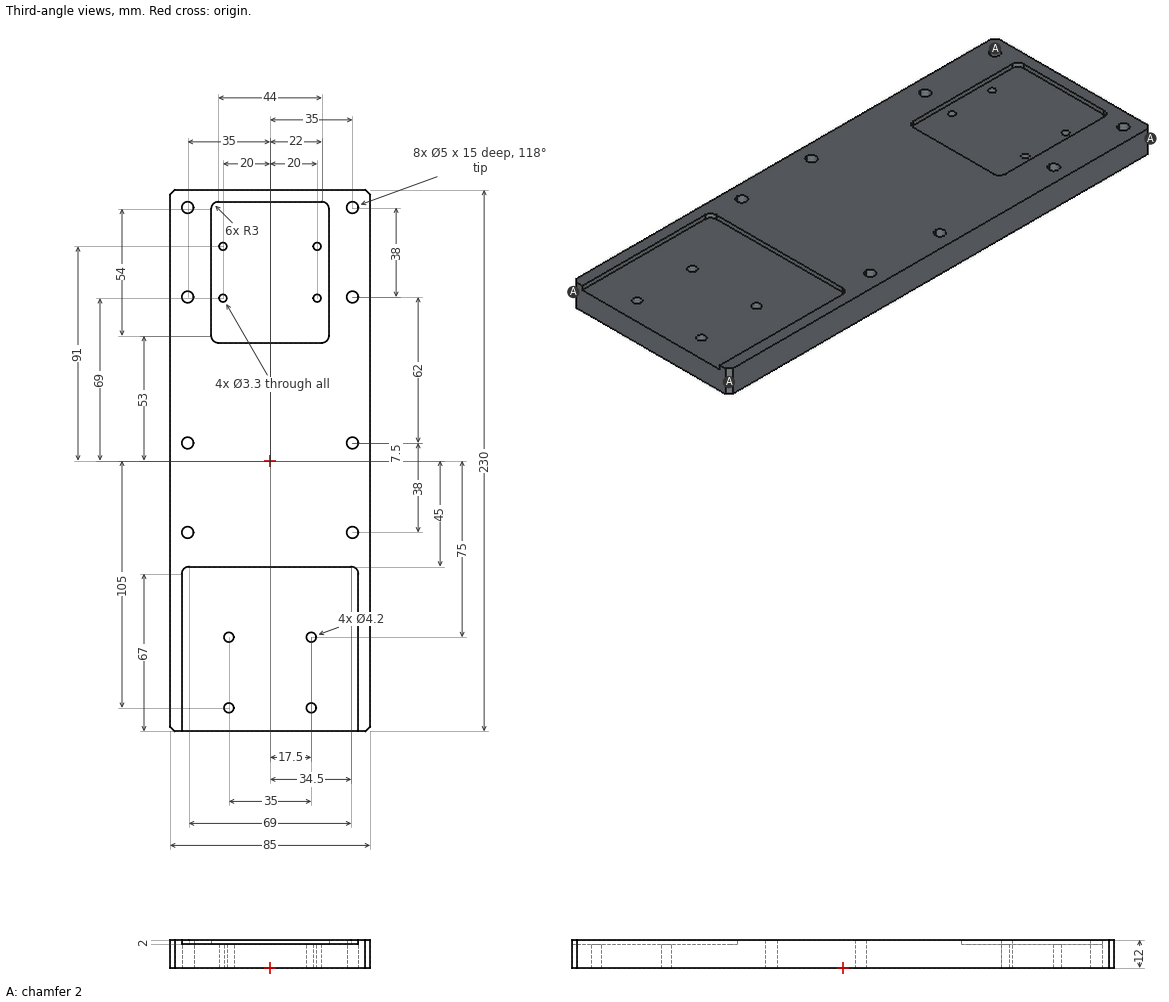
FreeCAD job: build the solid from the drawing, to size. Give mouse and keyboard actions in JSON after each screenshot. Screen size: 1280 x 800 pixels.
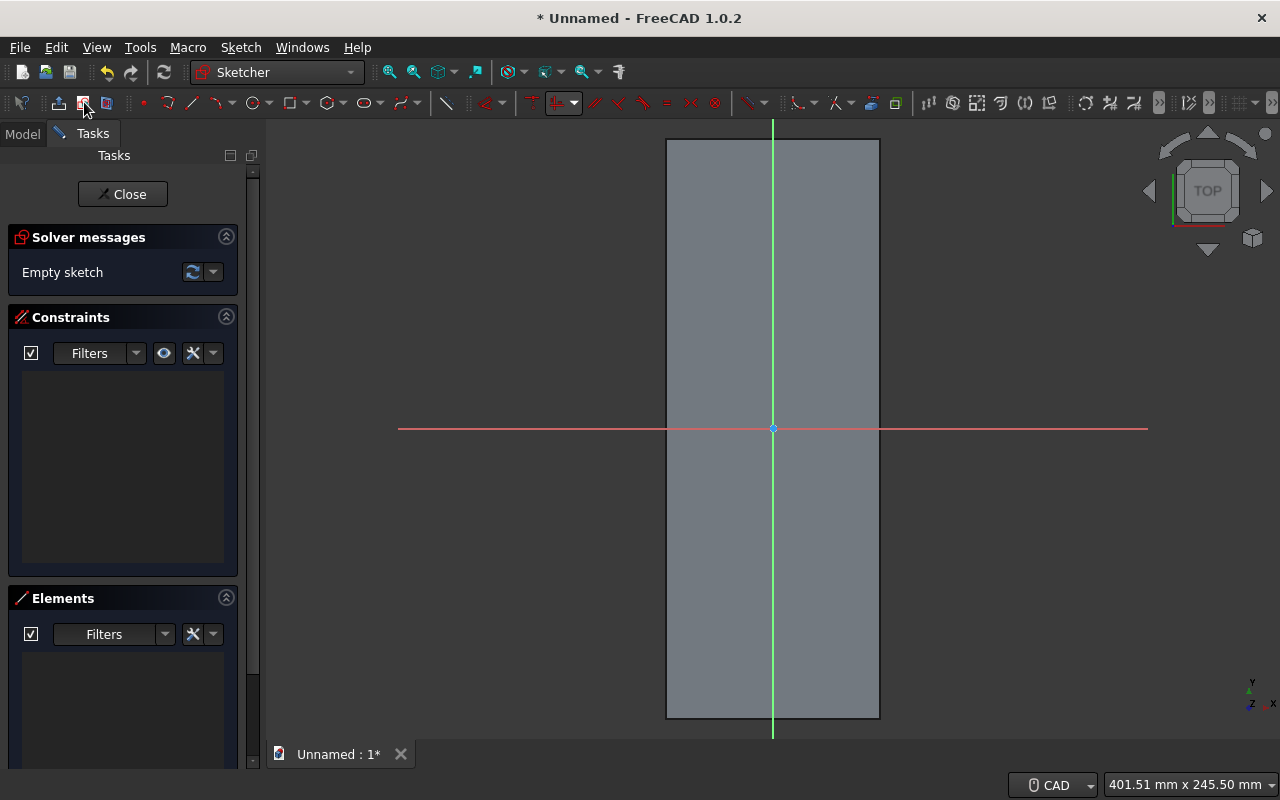
{"action": "scroll", "coordinate": [565, 416], "scroll_direction": "down", "scroll_amount": 2}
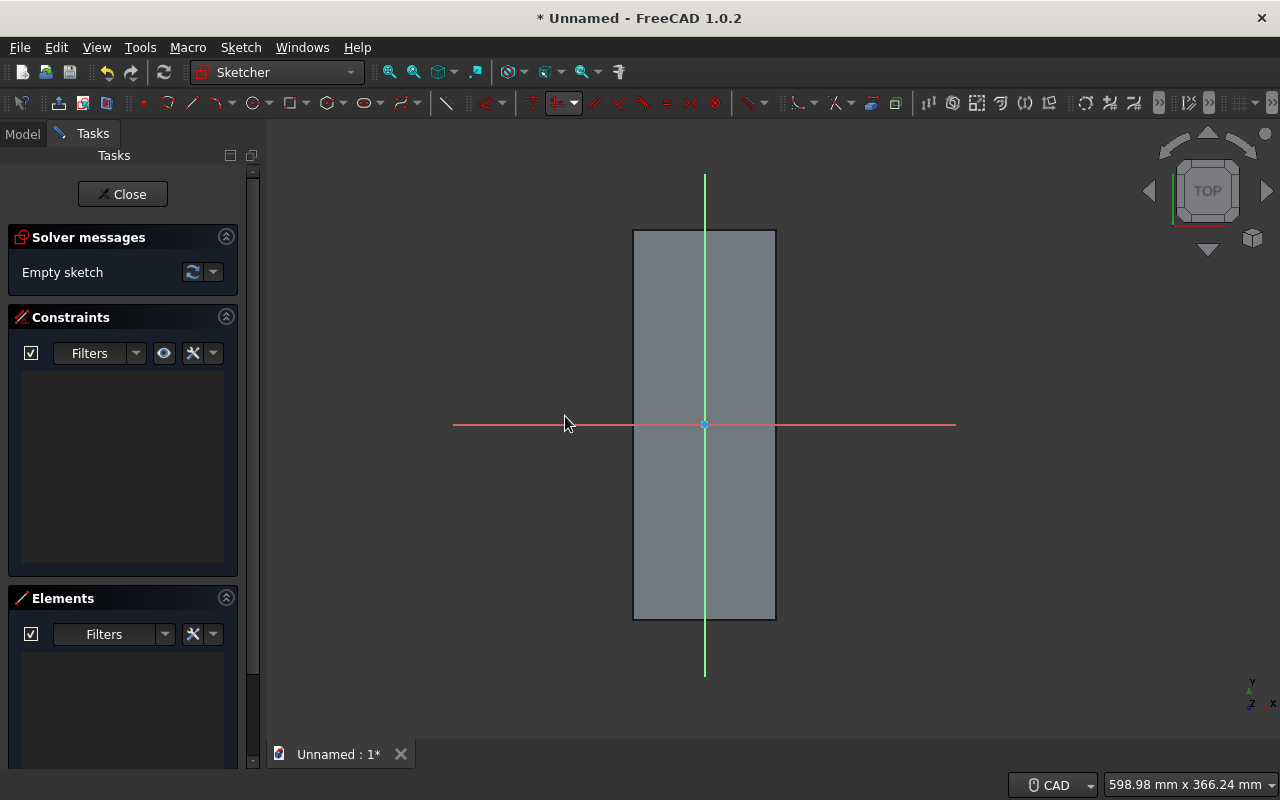
{"action": "key", "text": "g l"}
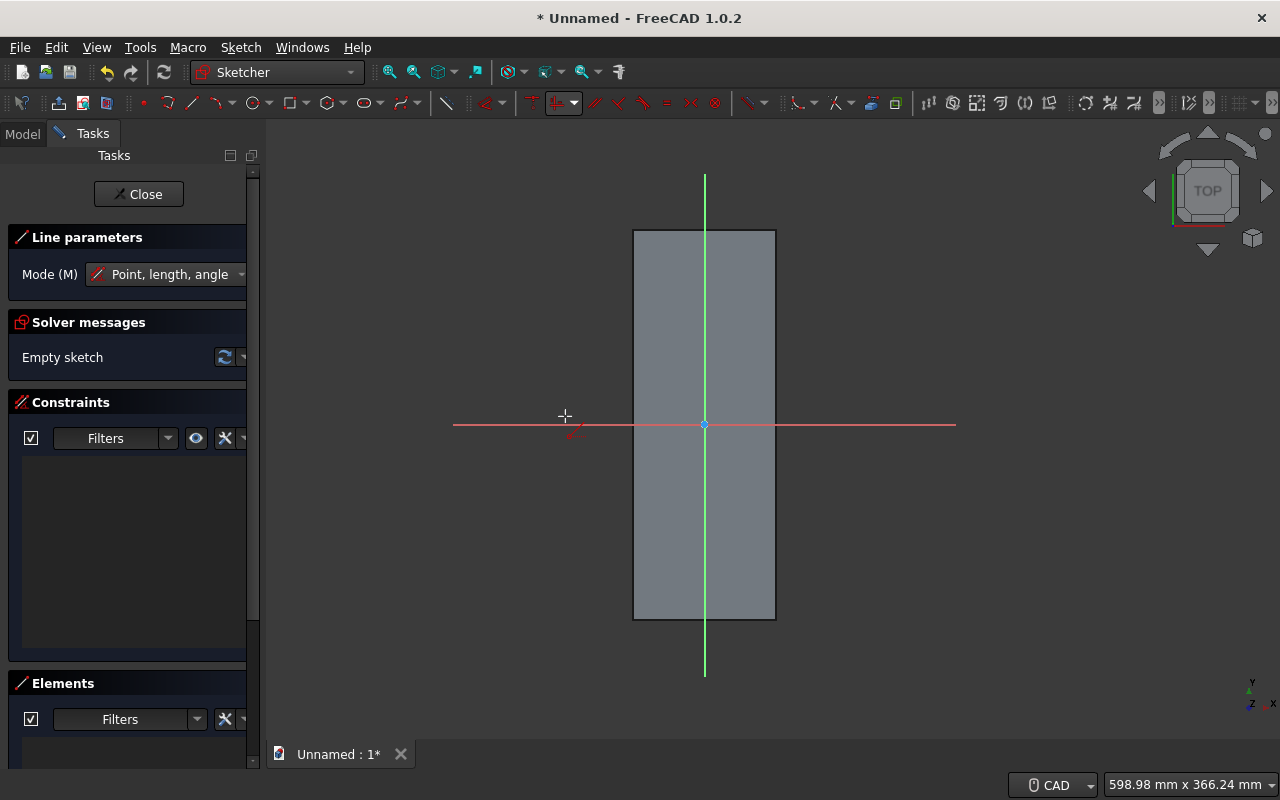
{"action": "left_click", "coordinate": [742, 239]}
{"action": "left_click", "coordinate": [667, 239]}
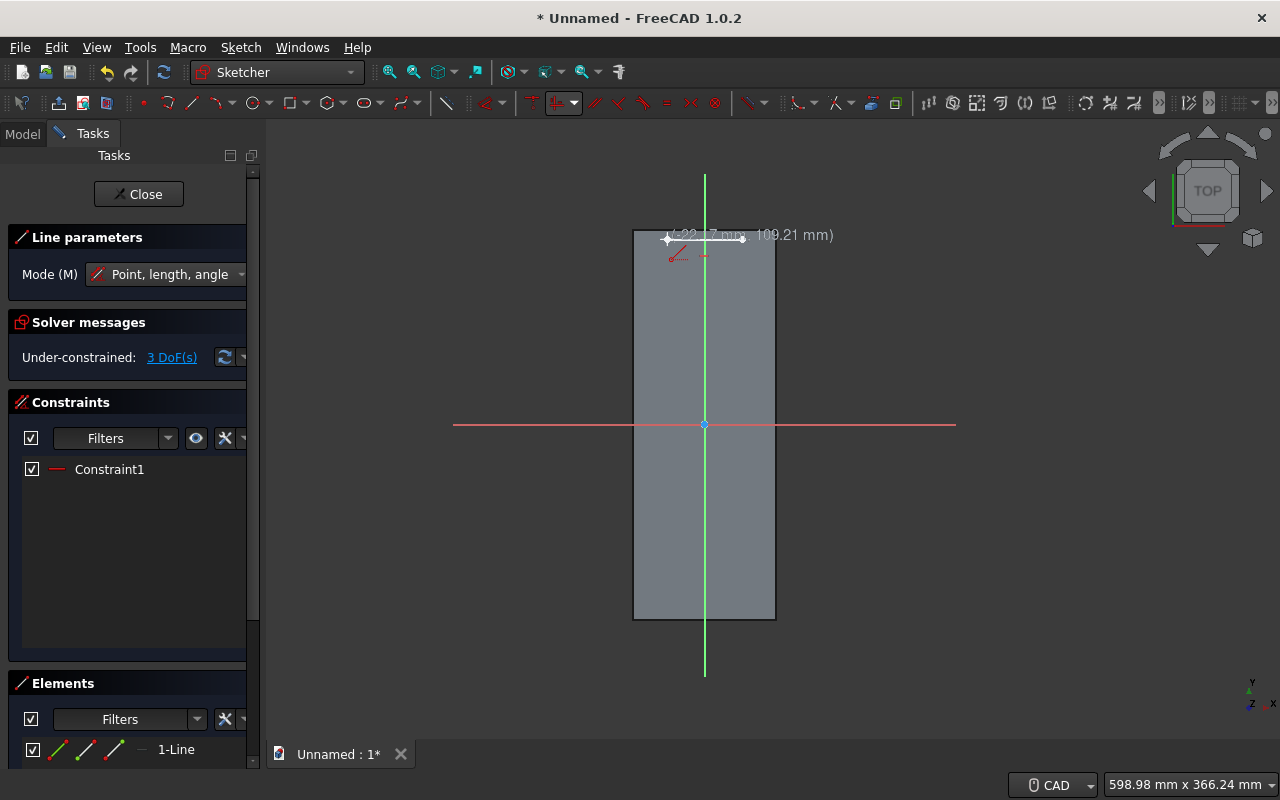
{"action": "scroll", "coordinate": [662, 244], "scroll_direction": "up", "scroll_amount": 4}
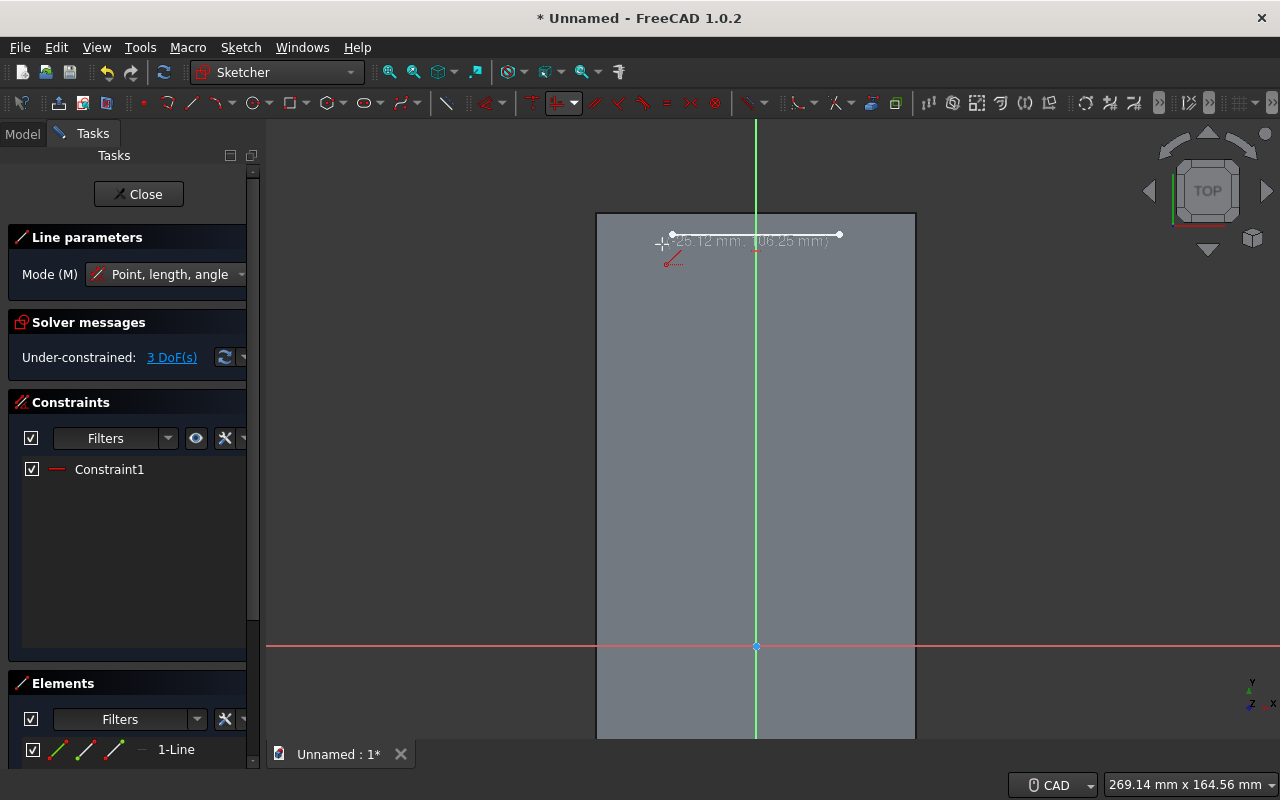
{"action": "left_click", "coordinate": [662, 243]}
{"action": "left_click", "coordinate": [662, 447]}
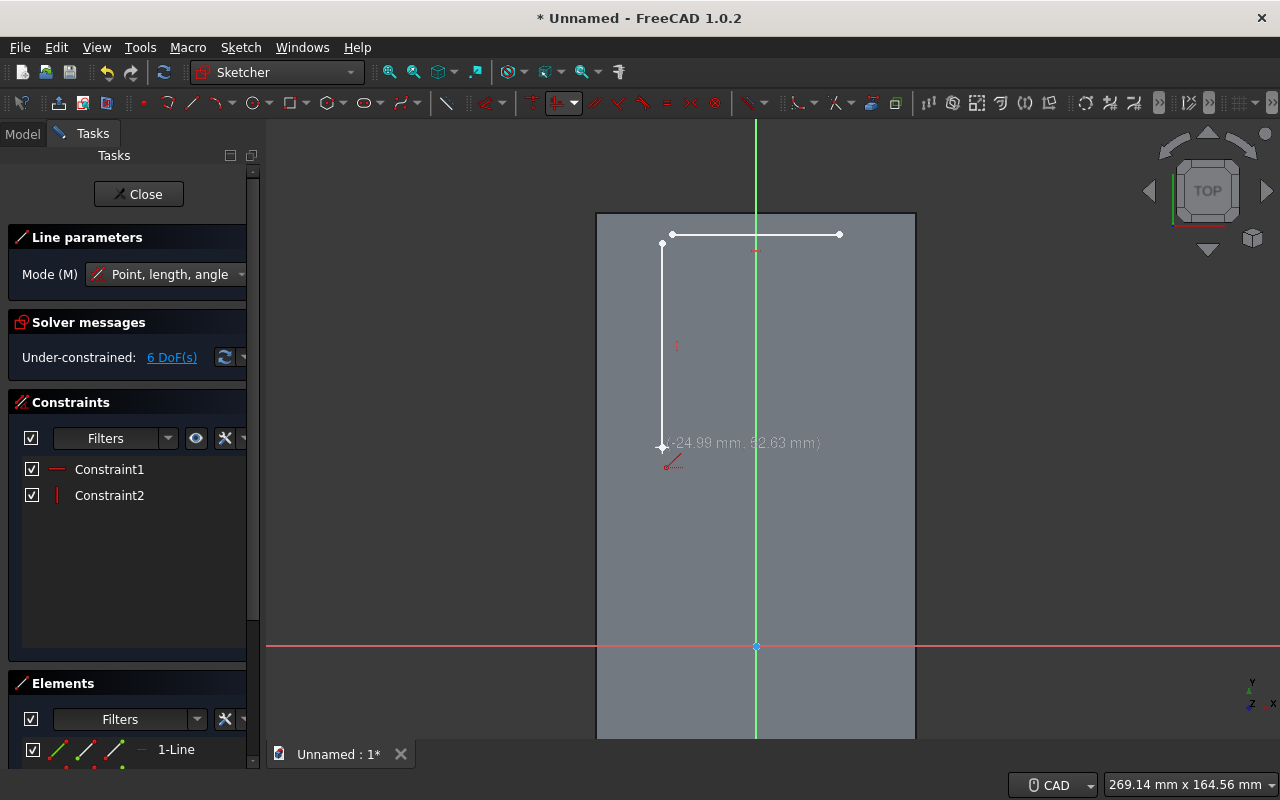
{"action": "left_click", "coordinate": [673, 458]}
{"action": "left_click", "coordinate": [839, 458]}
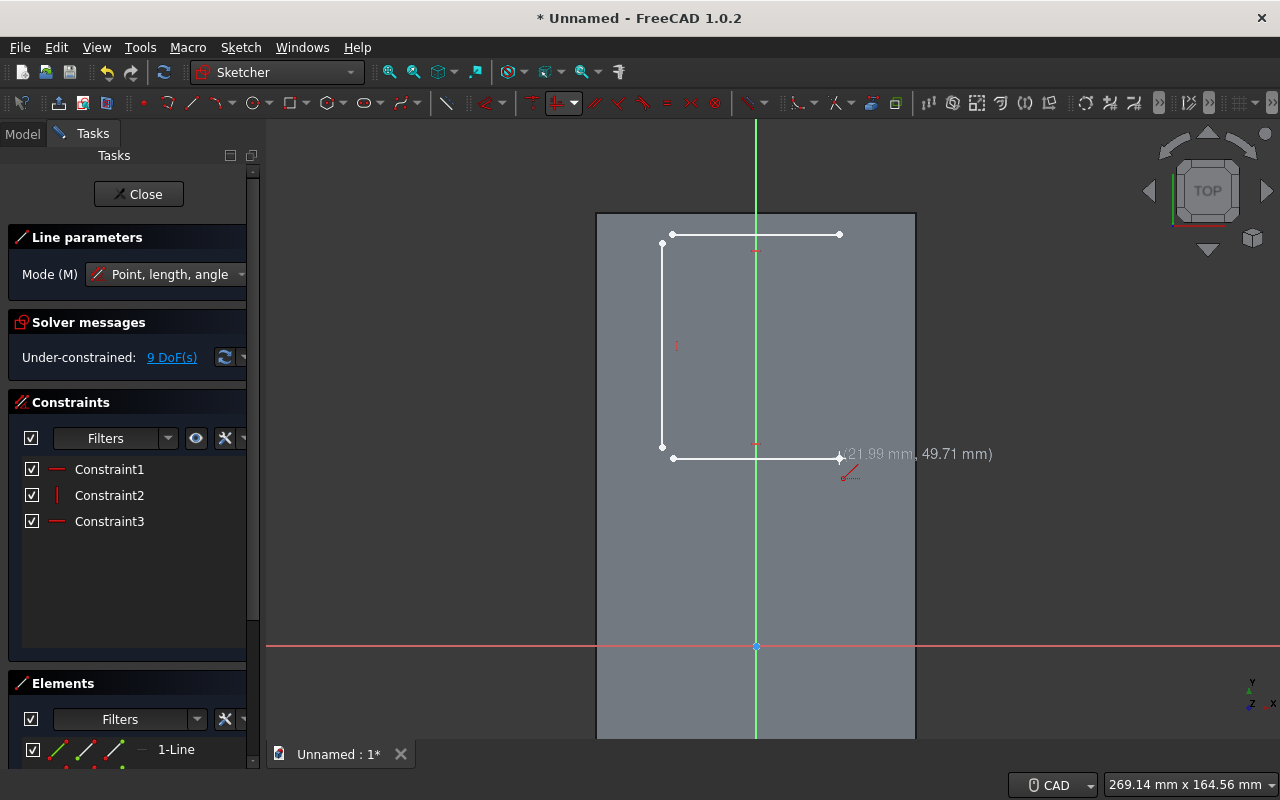
{"action": "left_click", "coordinate": [850, 447]}
{"action": "left_click", "coordinate": [850, 243]}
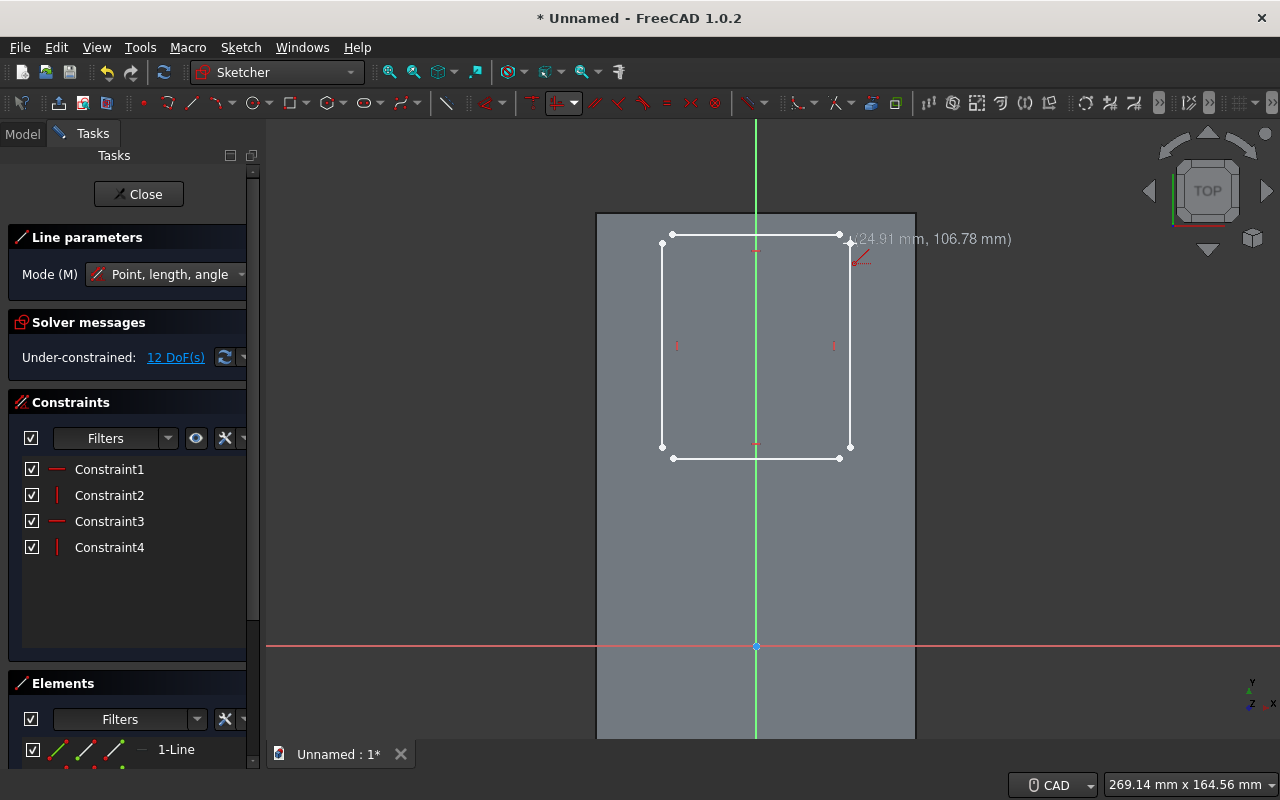
{"action": "key", "text": "g 3 a"}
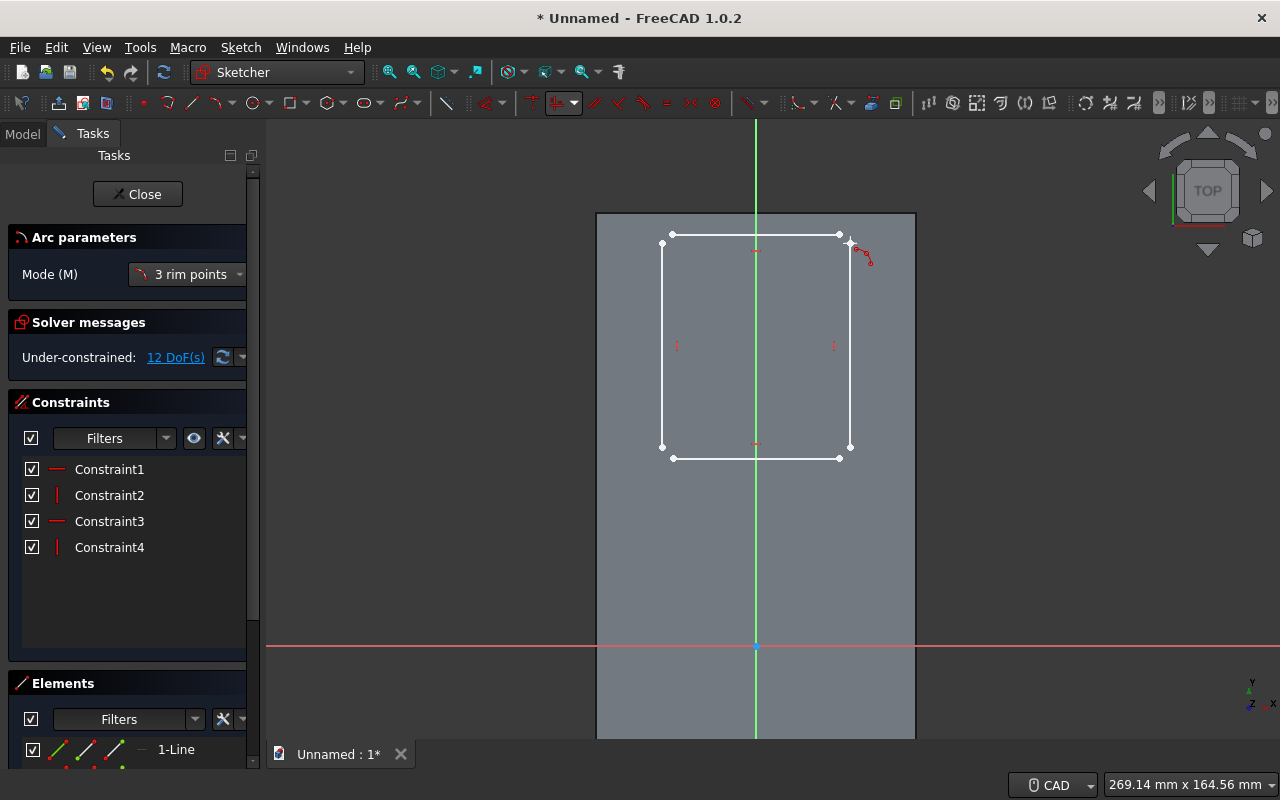
{"action": "left_click", "coordinate": [673, 235]}
{"action": "left_click", "coordinate": [662, 244]}